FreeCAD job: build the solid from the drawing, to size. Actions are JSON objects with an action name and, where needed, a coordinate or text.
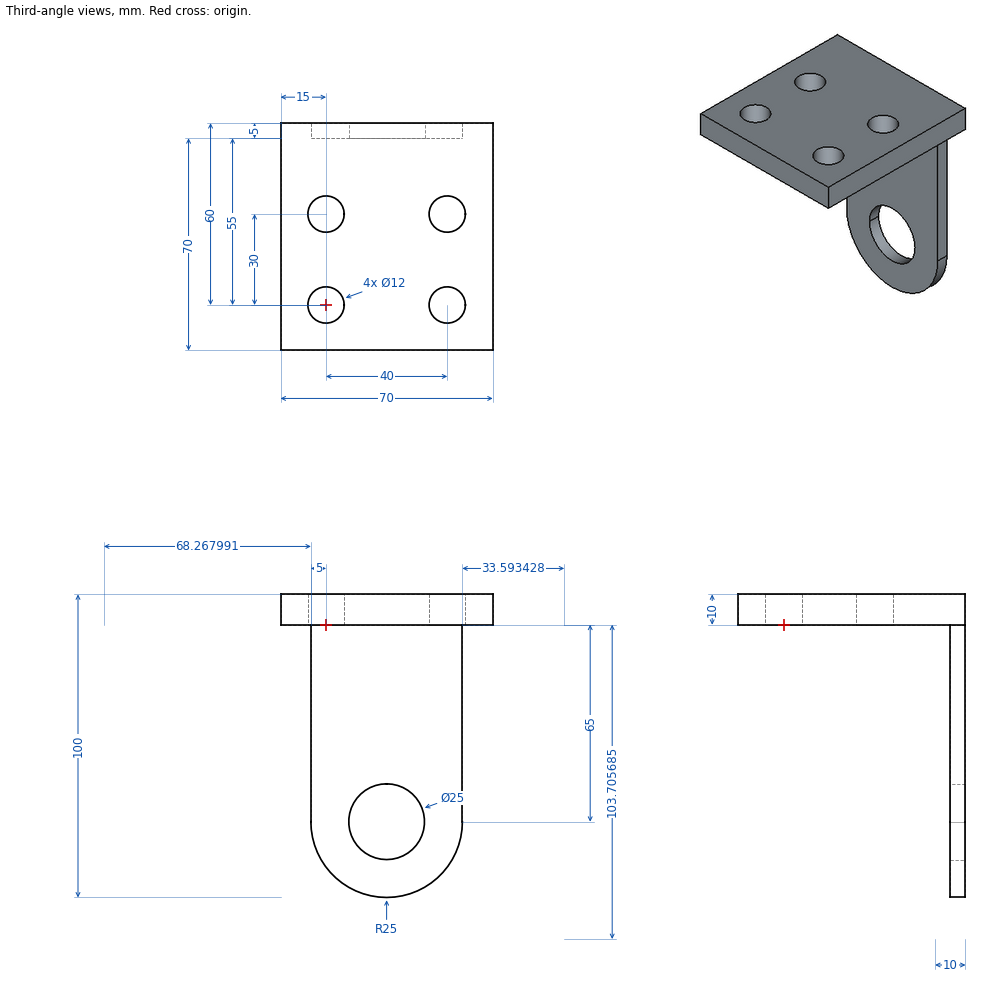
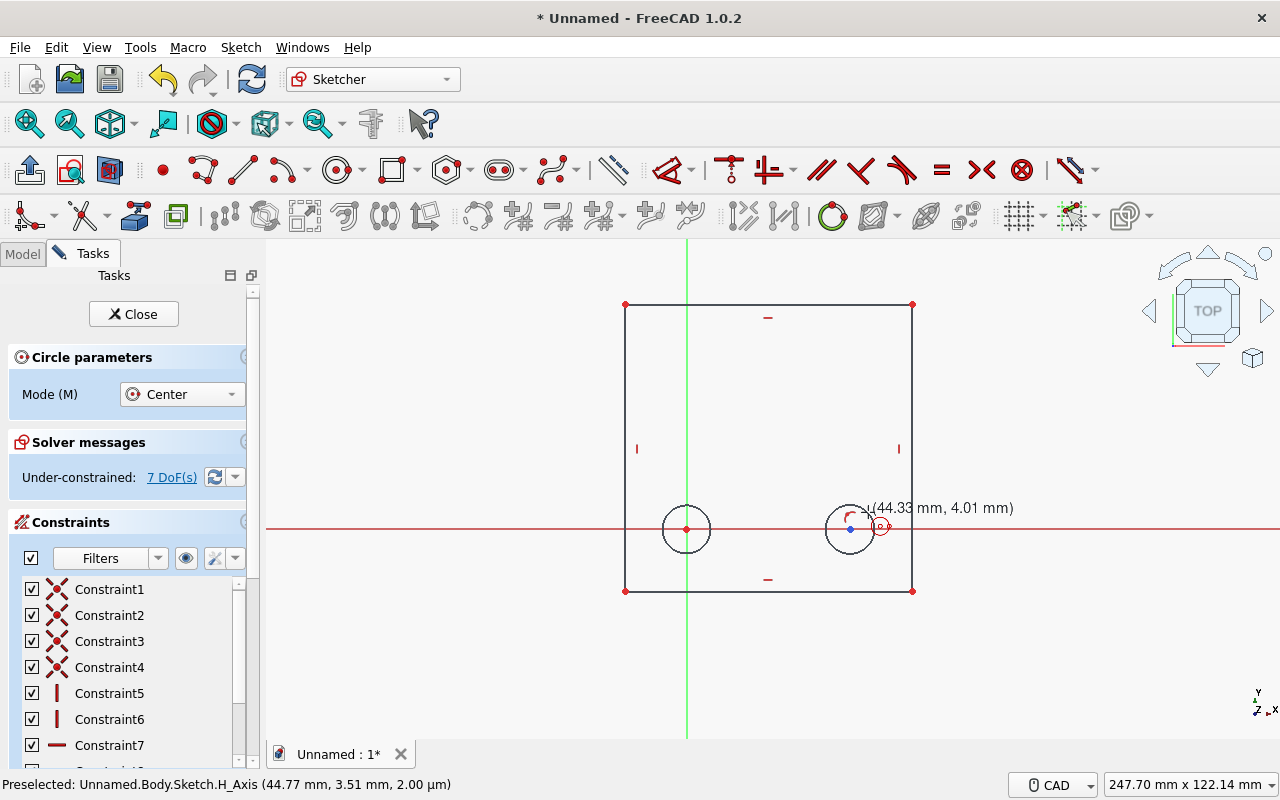
{"action": "left_click", "coordinate": [687, 407]}
{"action": "left_click", "coordinate": [704, 389]}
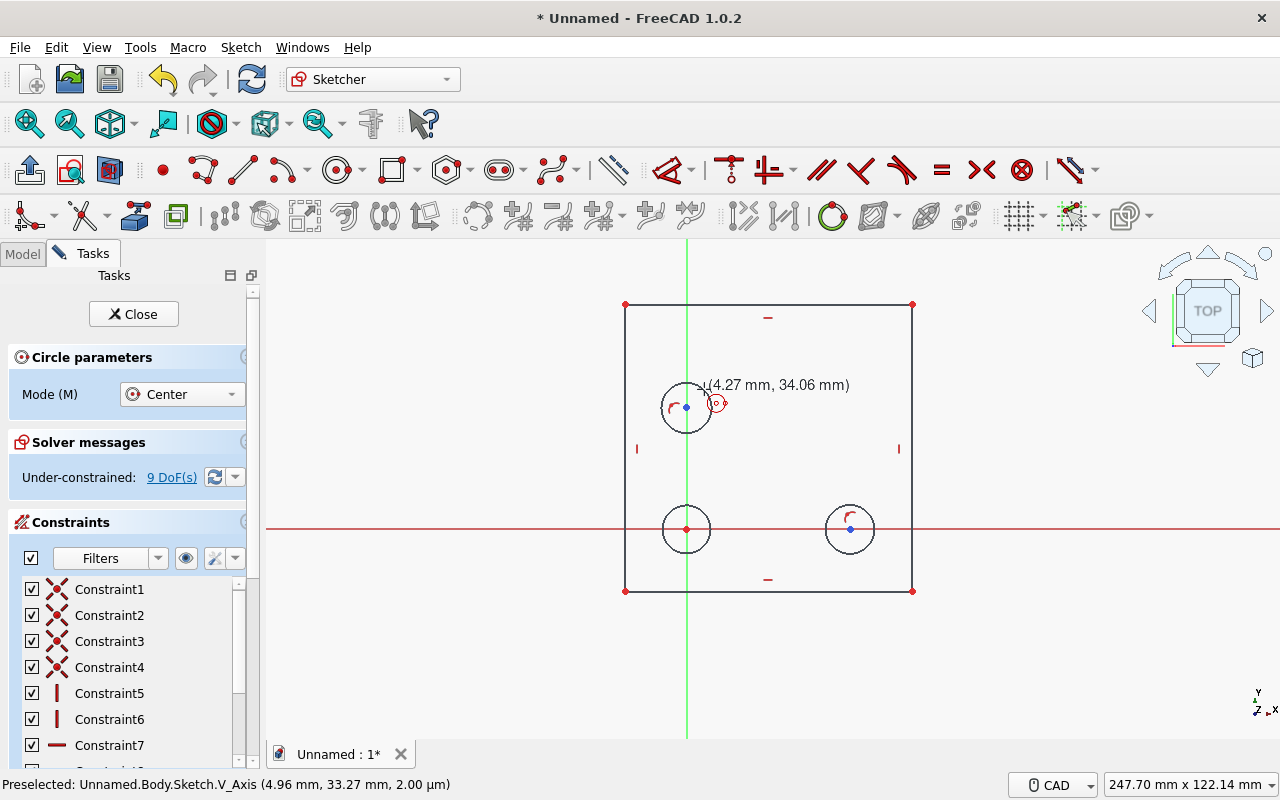
{"action": "left_click", "coordinate": [850, 407]}
{"action": "left_click", "coordinate": [868, 389]}
{"action": "key", "text": "Escape"}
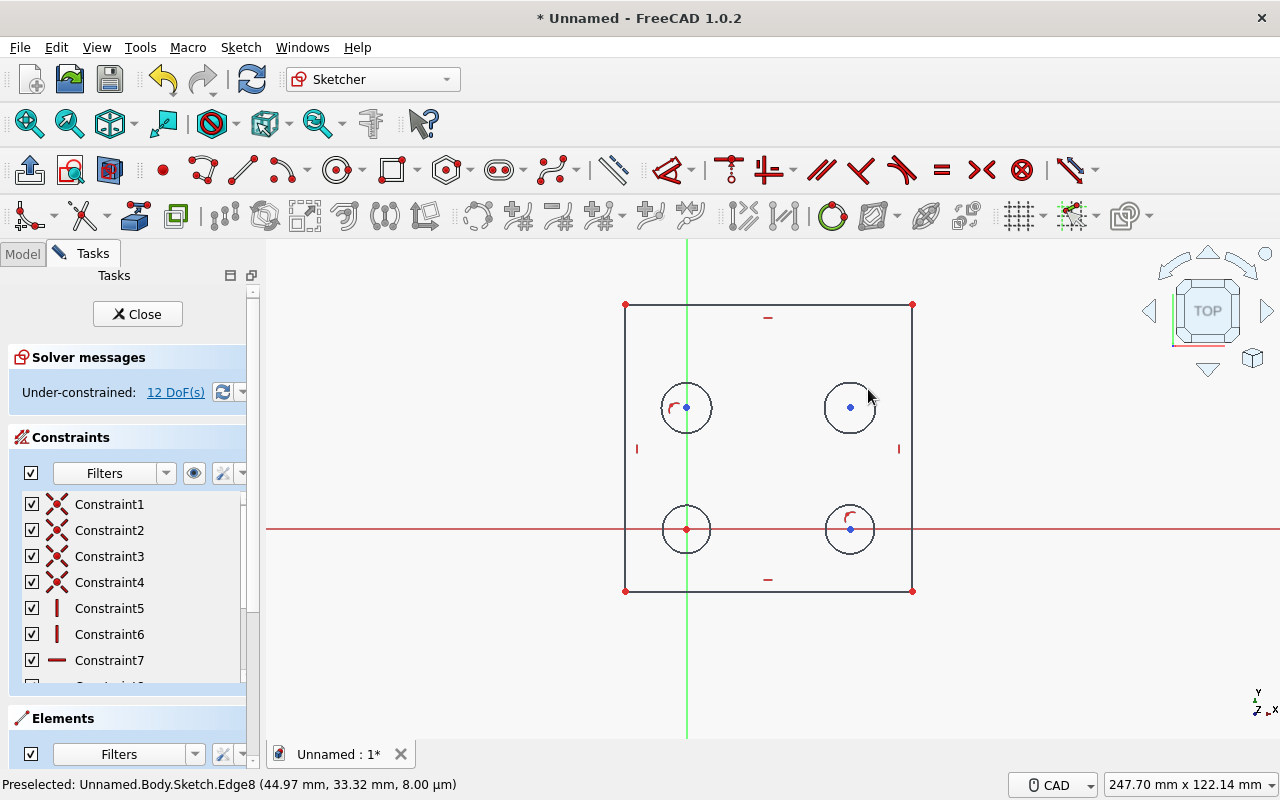
{"action": "left_click", "coordinate": [703, 512]}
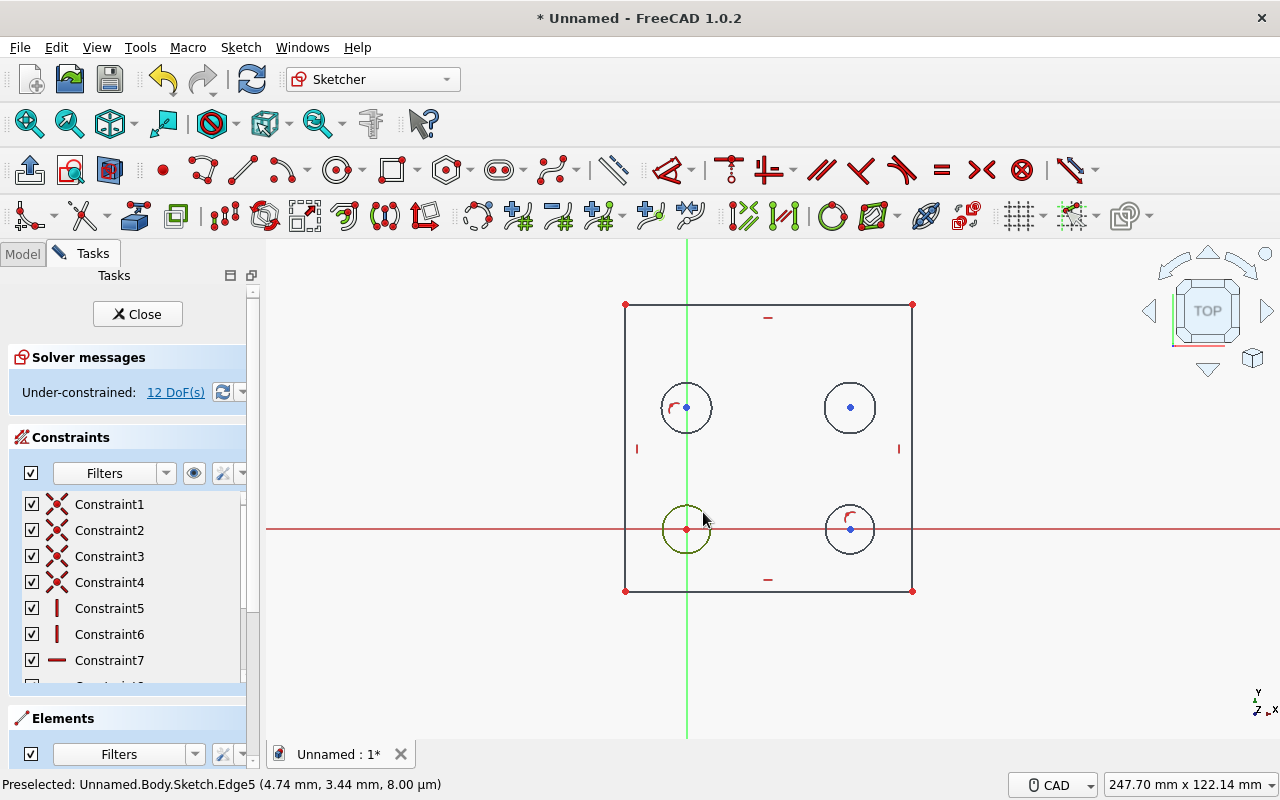
{"action": "left_click", "coordinate": [867, 512]}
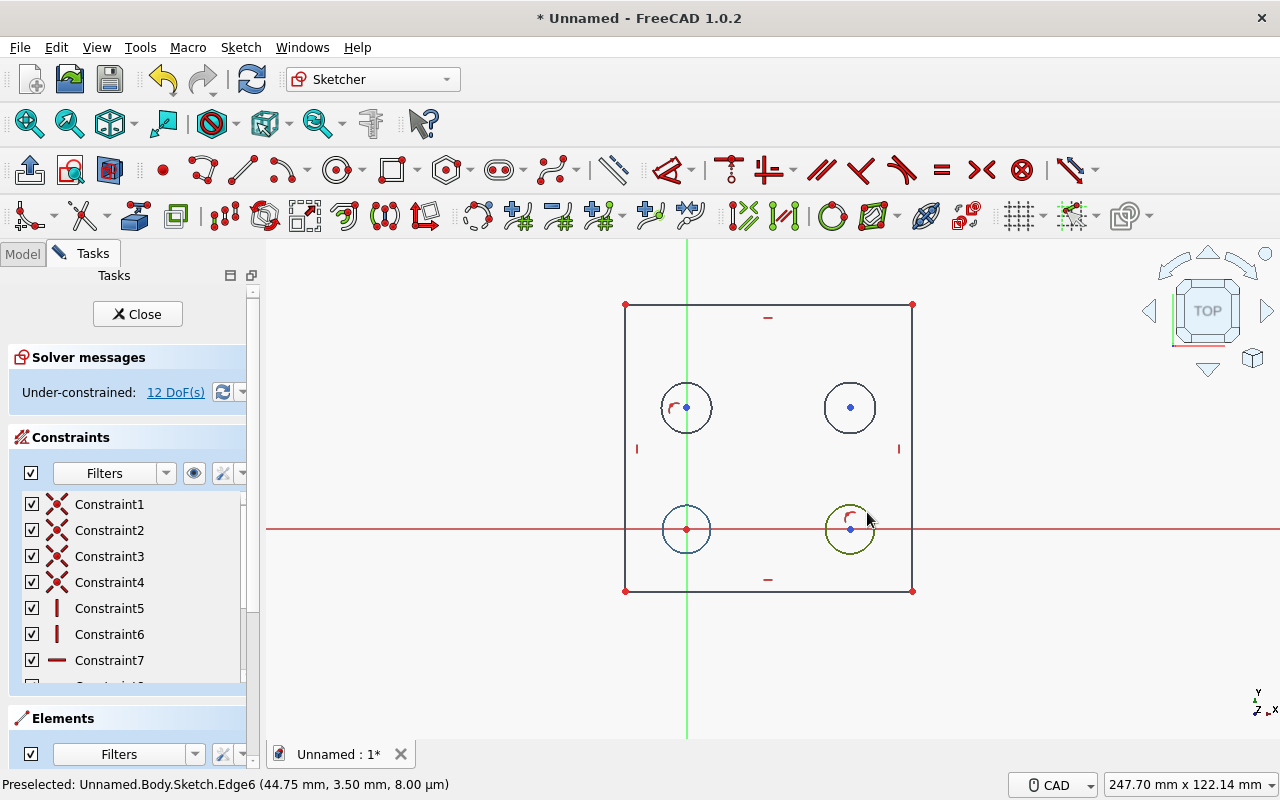
{"action": "left_click", "coordinate": [704, 390]}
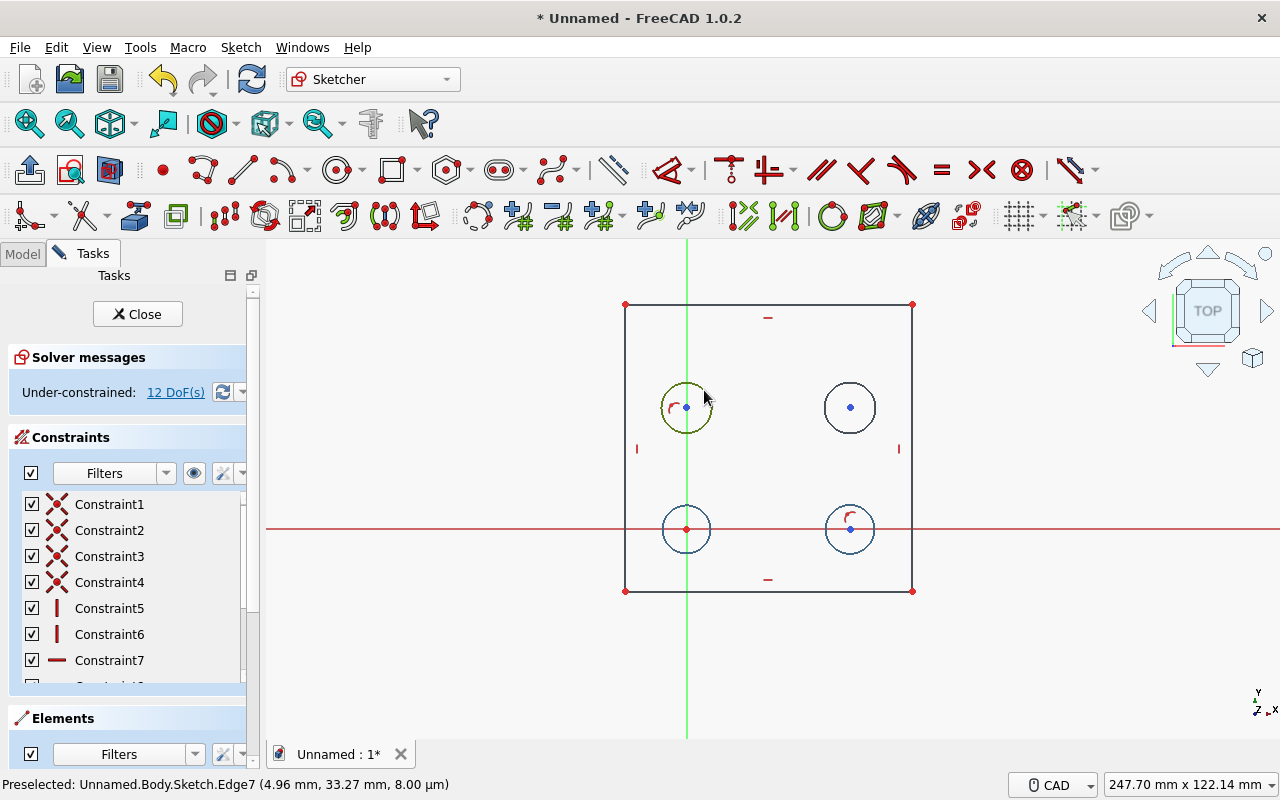
{"action": "left_click", "coordinate": [868, 390]}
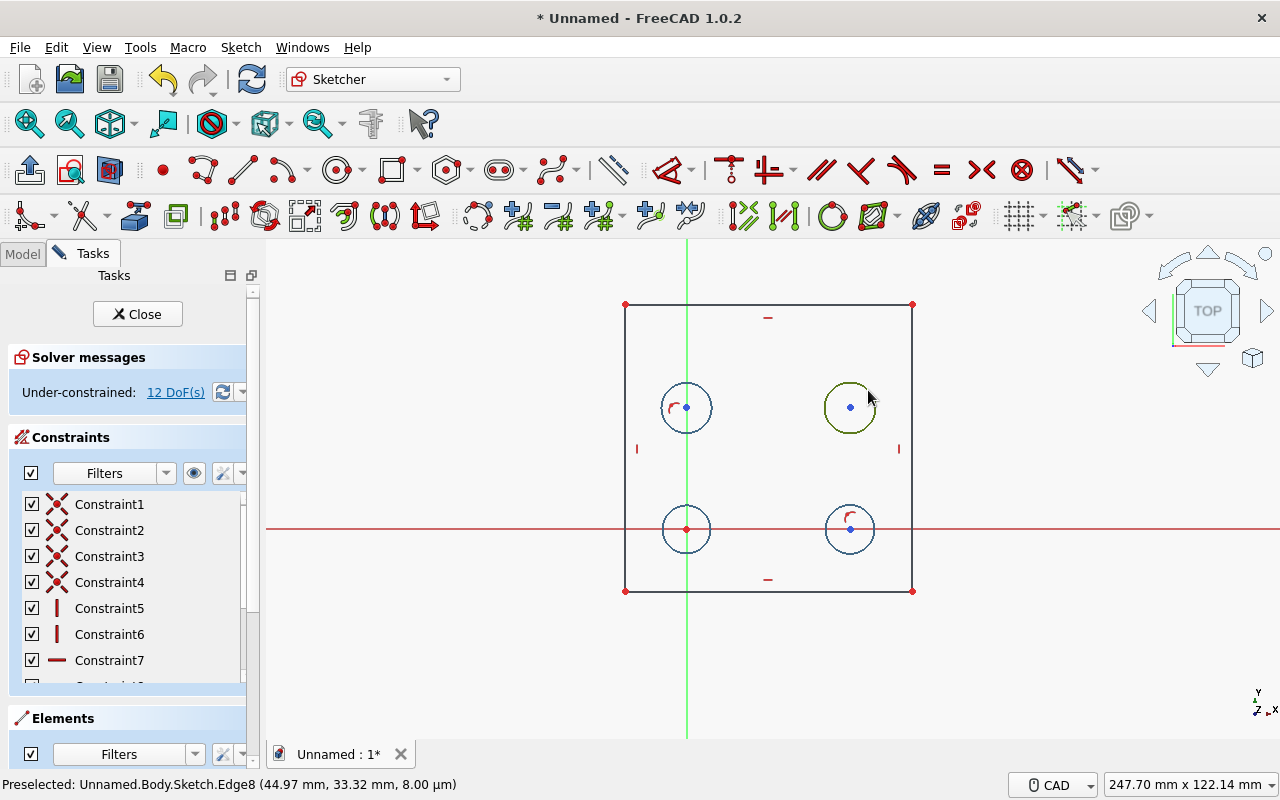
{"action": "left_click", "coordinate": [942, 170]}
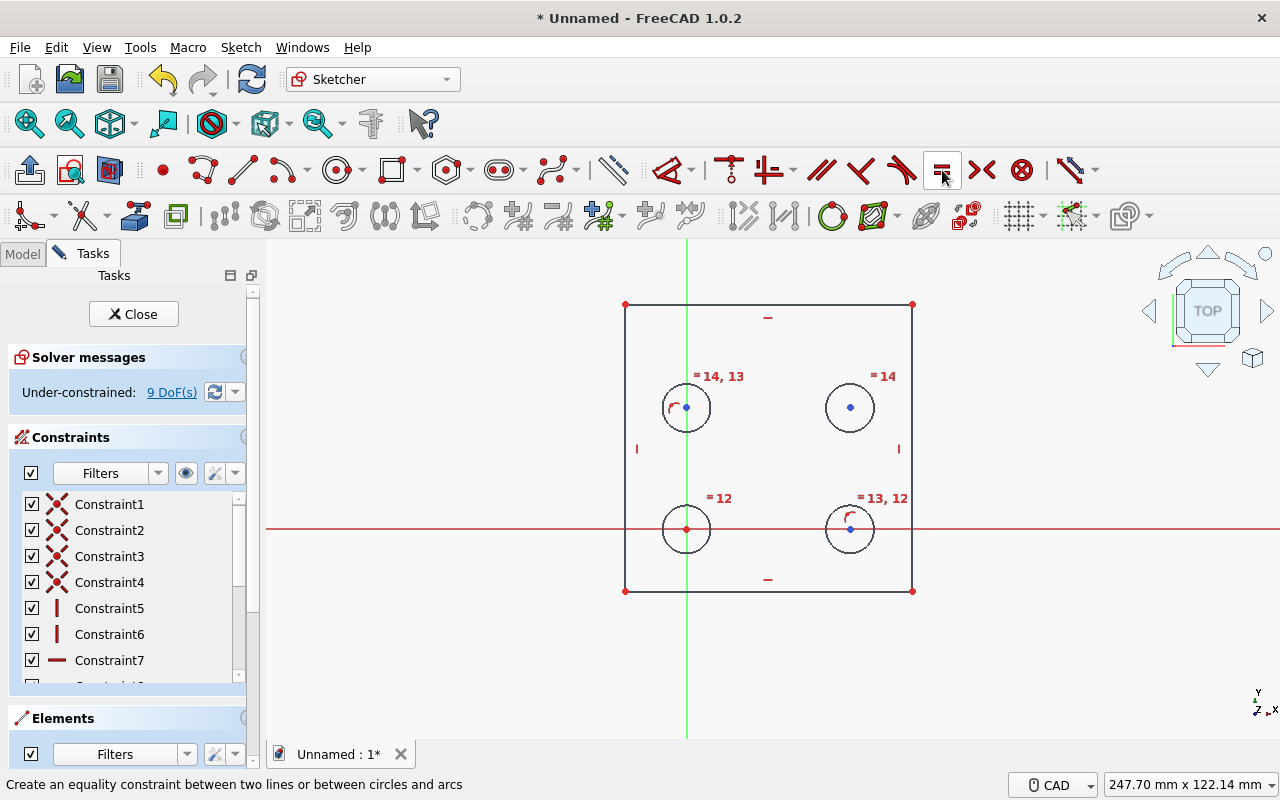
{"action": "left_click", "coordinate": [668, 170]}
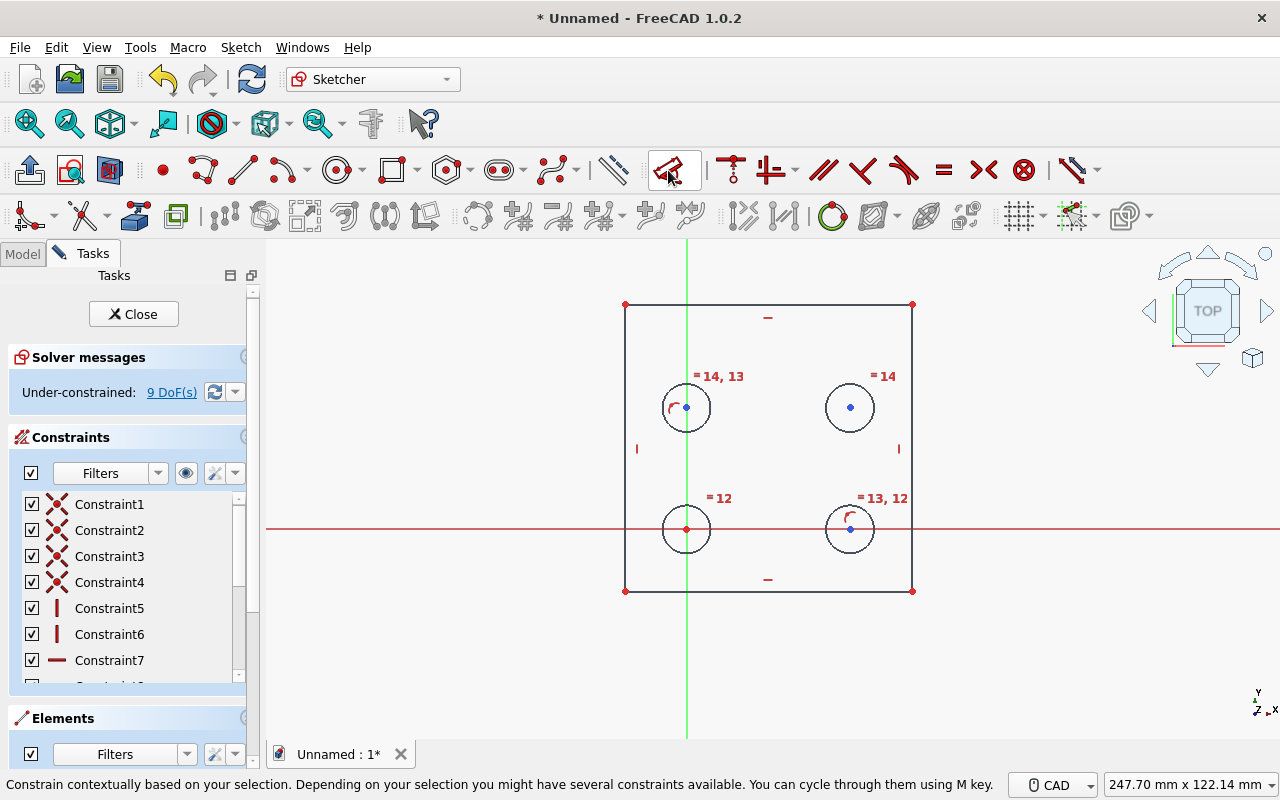
{"action": "left_click", "coordinate": [703, 512]}
{"action": "left_click", "coordinate": [725, 489]}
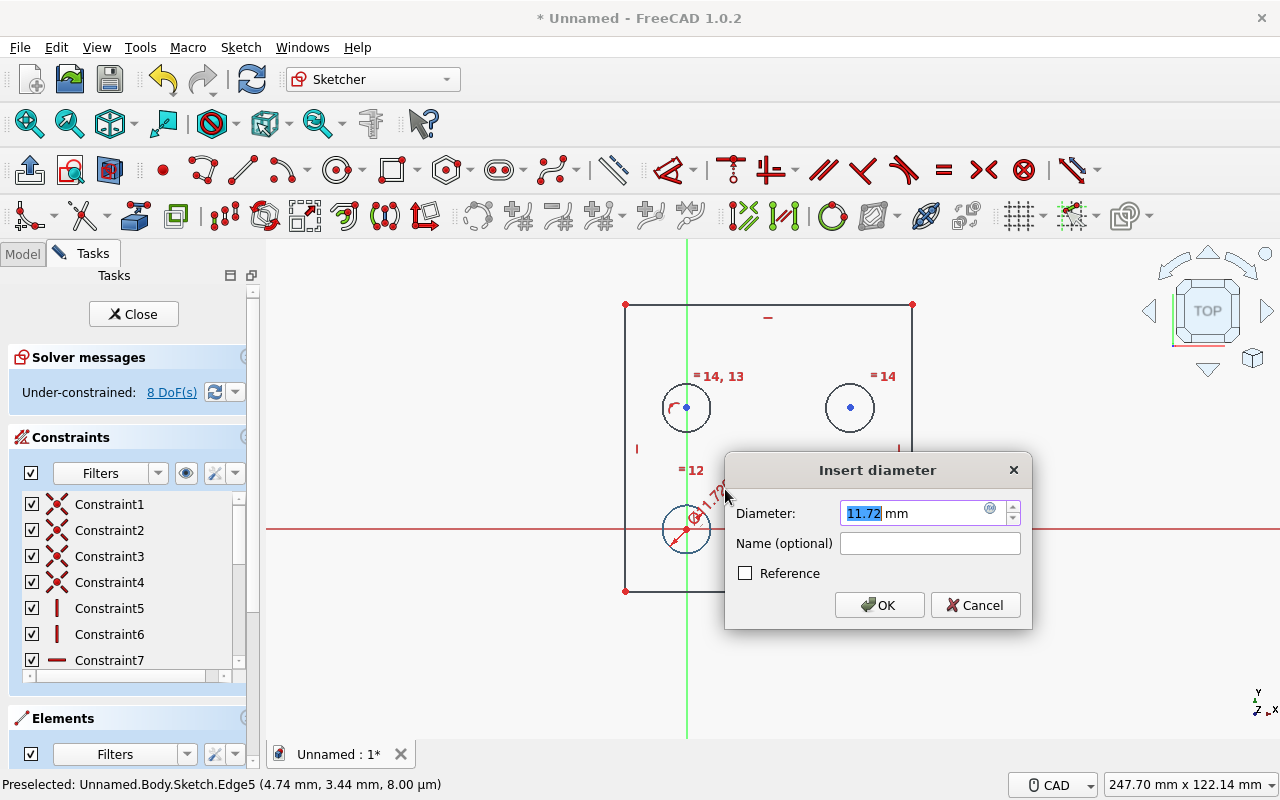
{"action": "type", "text": "12"}
{"action": "key", "text": "Return"}